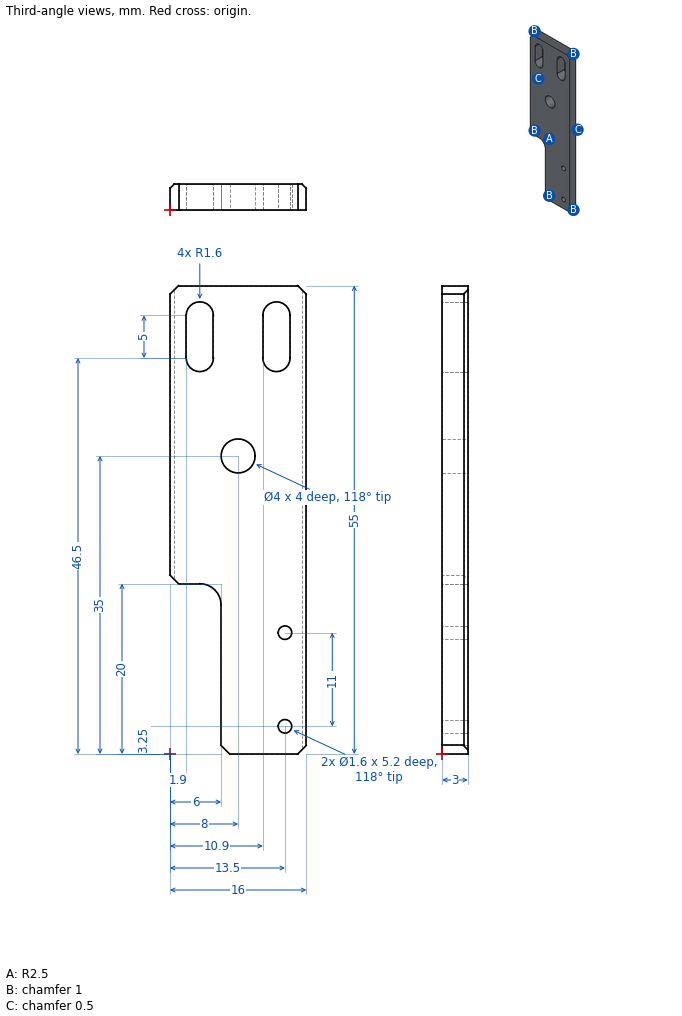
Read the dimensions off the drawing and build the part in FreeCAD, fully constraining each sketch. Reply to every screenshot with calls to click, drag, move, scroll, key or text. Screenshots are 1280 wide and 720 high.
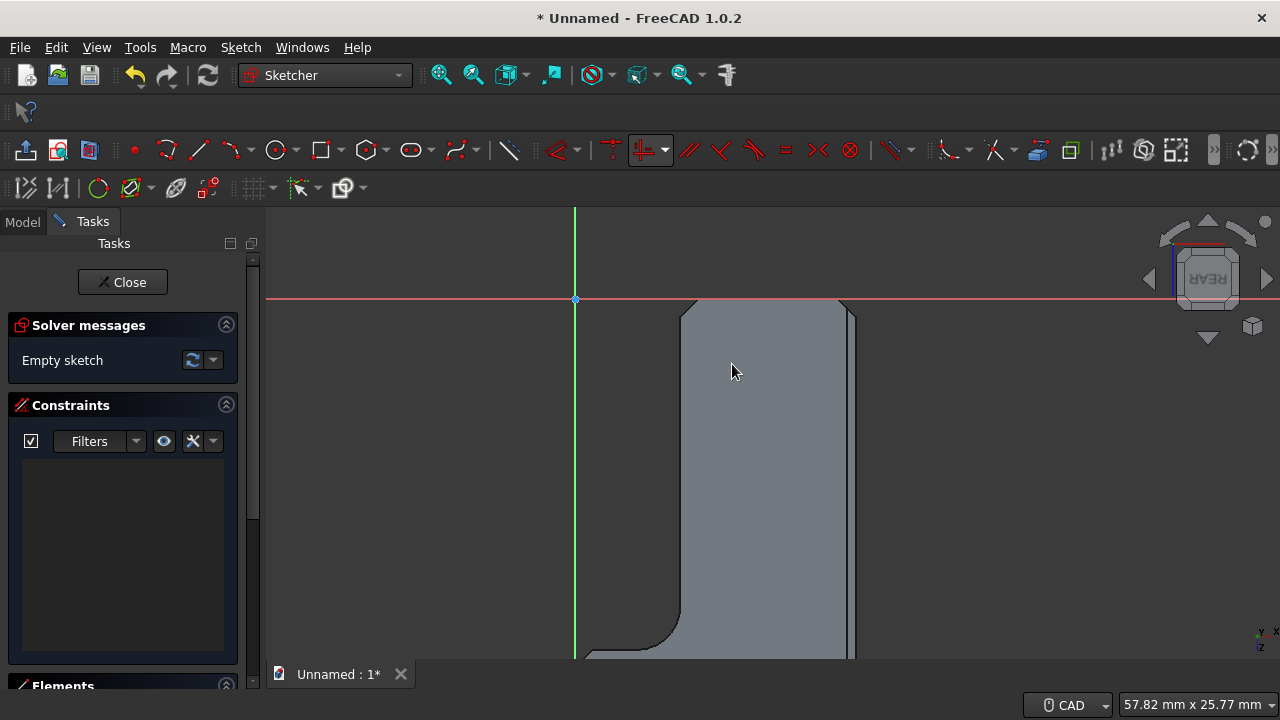
click(276, 150)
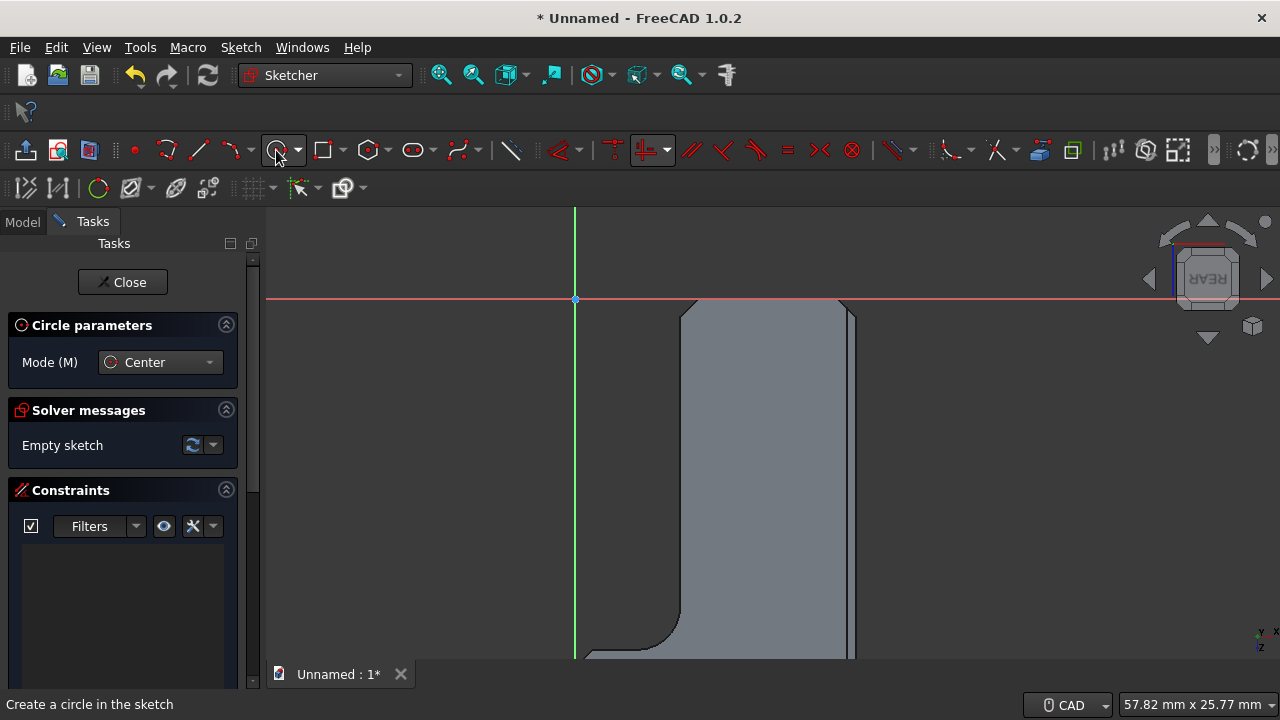
scroll(812, 356, up, 3)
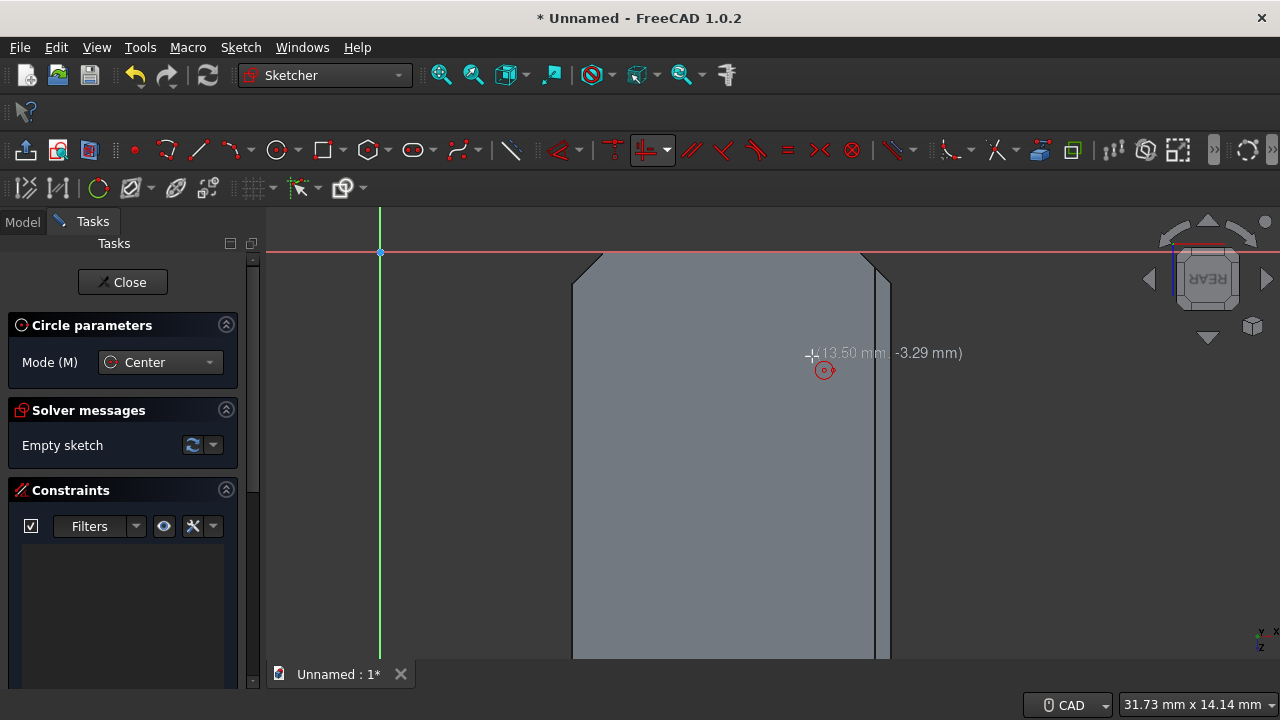
click(811, 356)
move(830, 338)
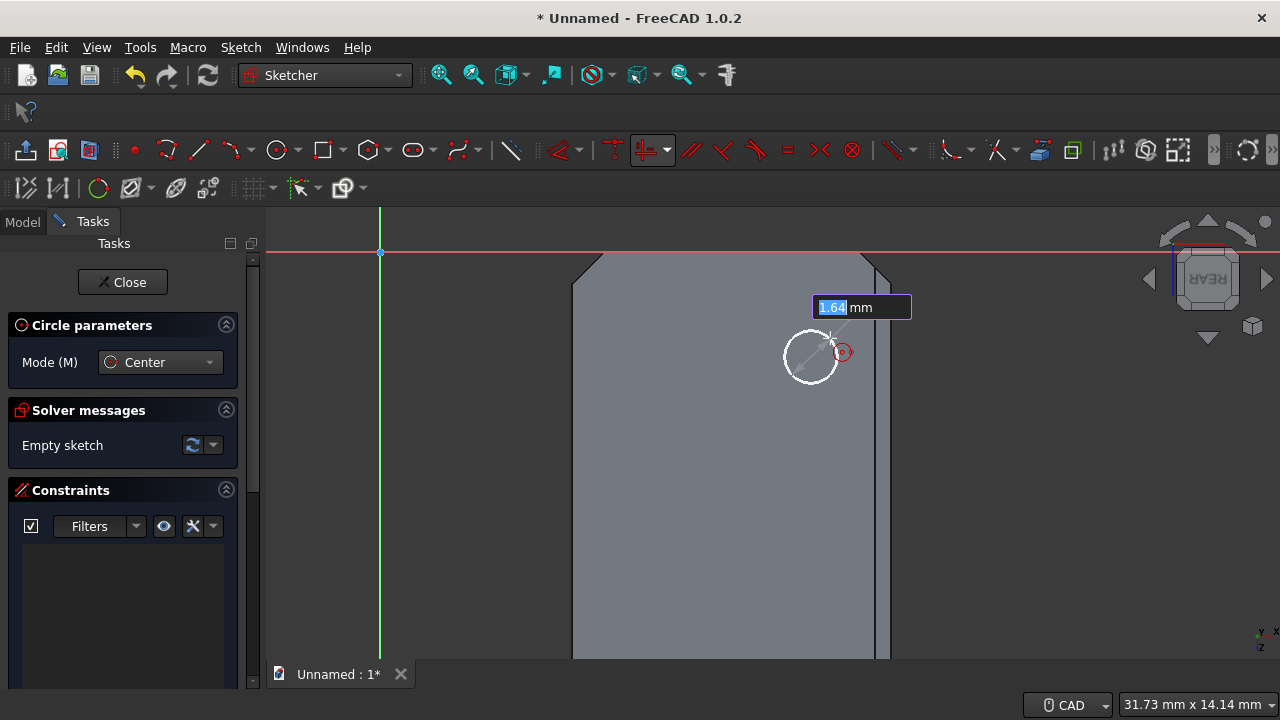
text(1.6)
key(Return)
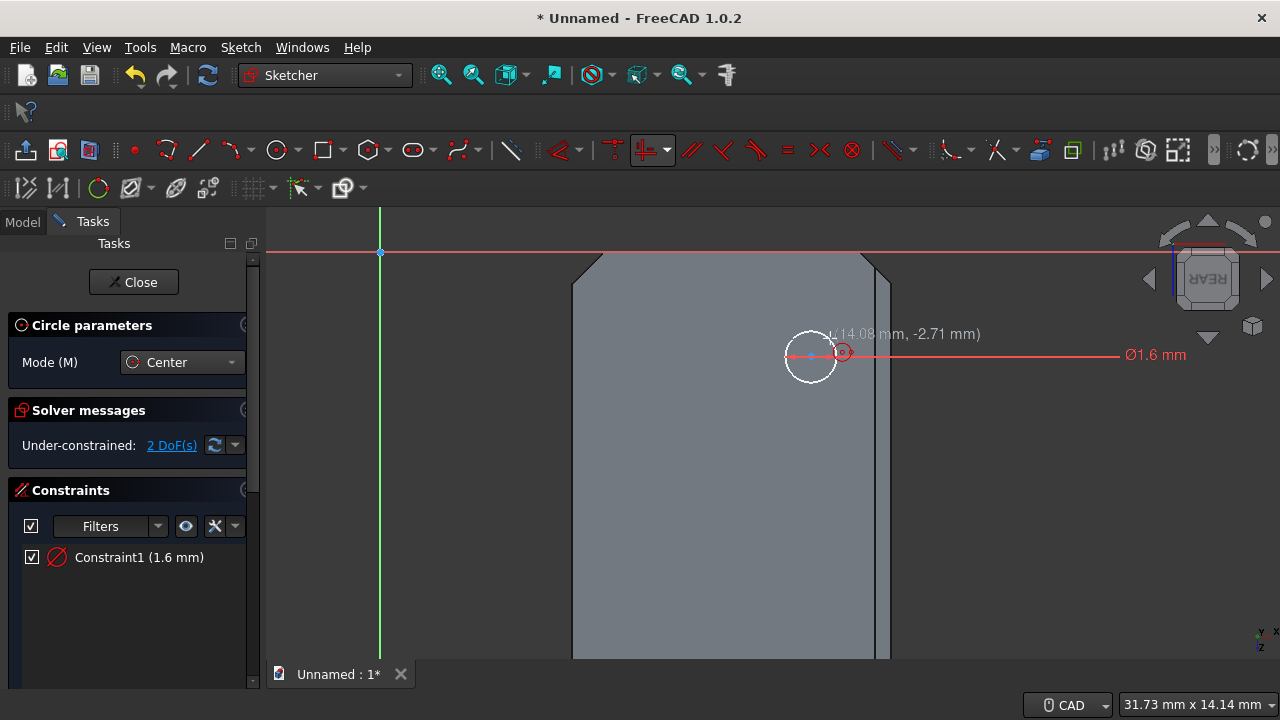
scroll(821, 360, down, 3)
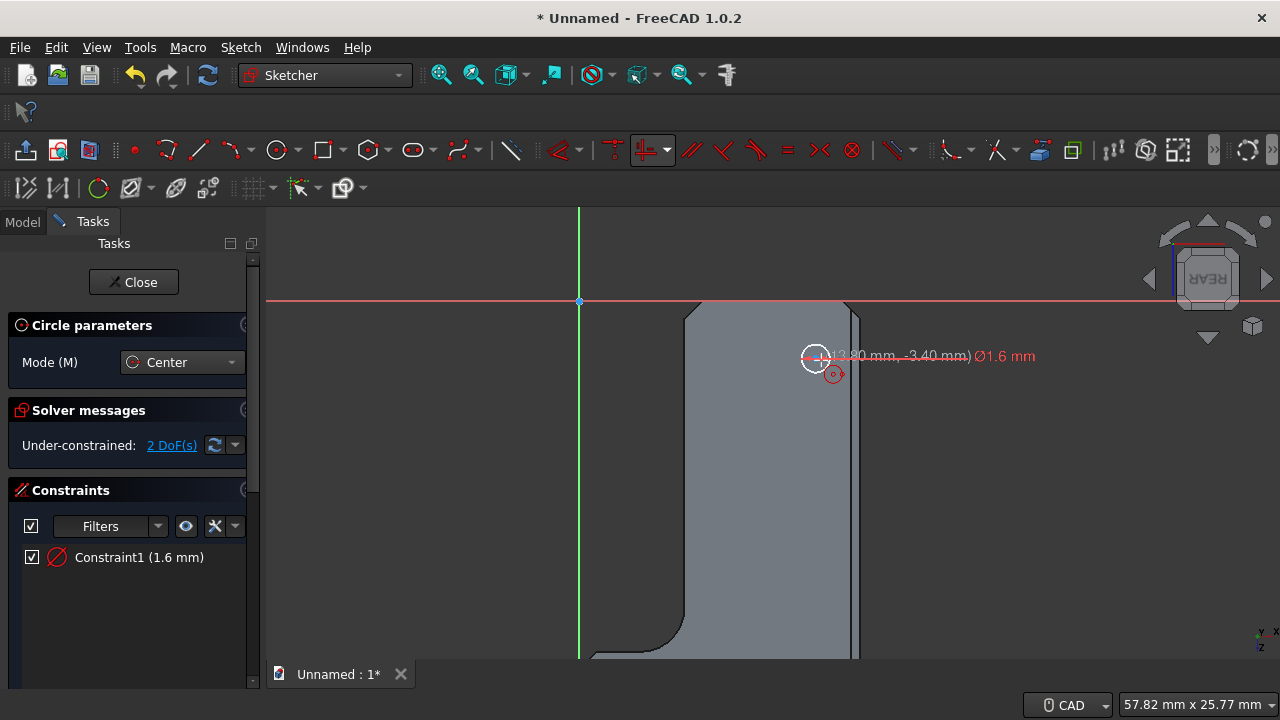
scroll(816, 551, up, 3)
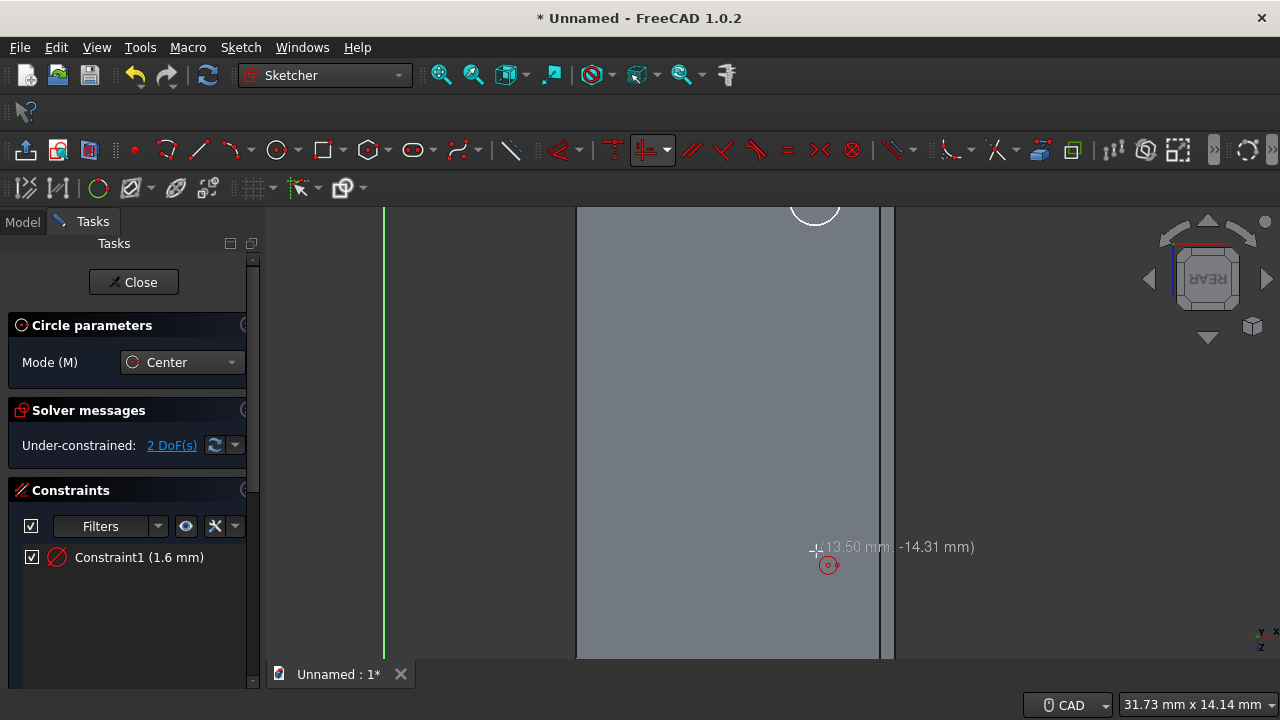
click(816, 550)
move(834, 532)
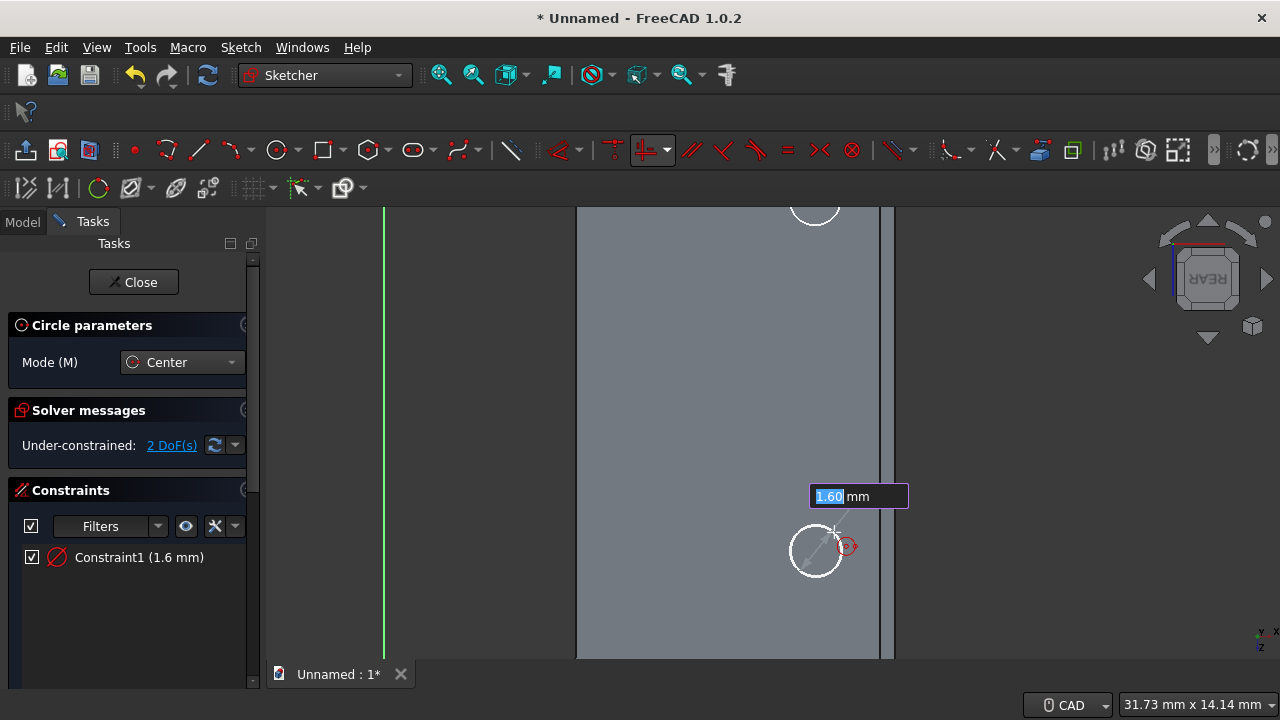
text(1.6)
key(Return)
key(Escape)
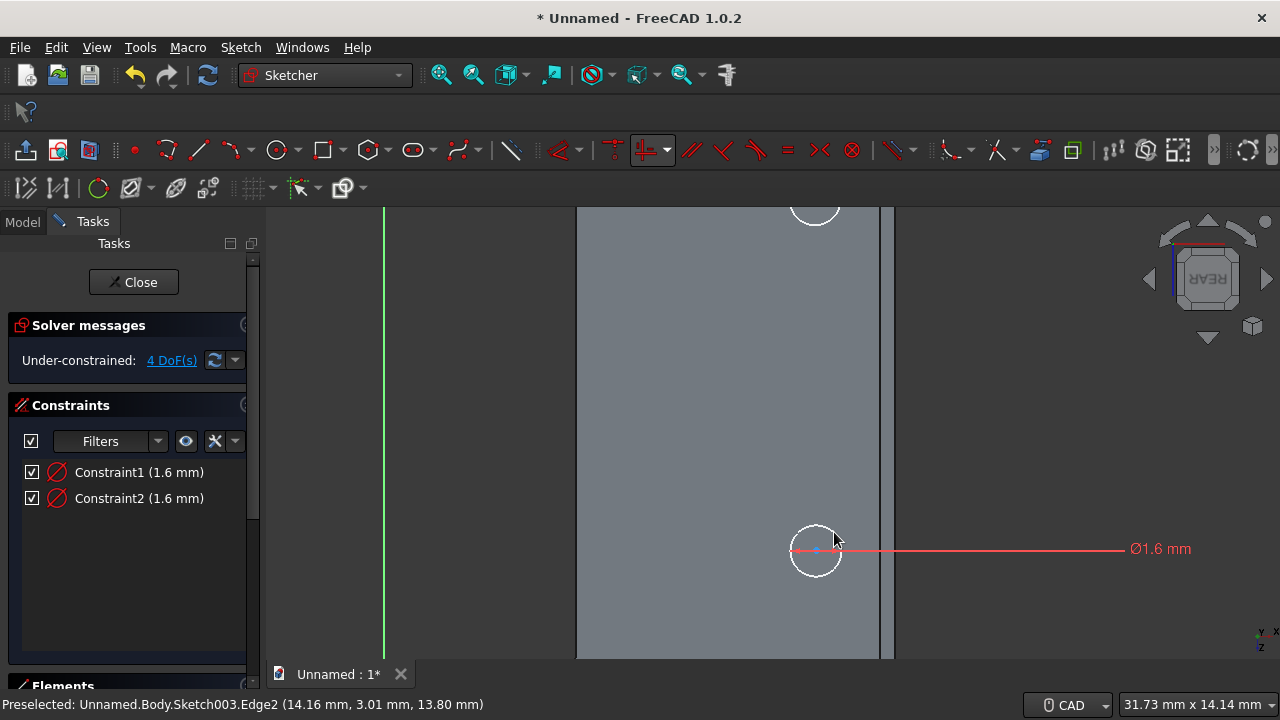
click(558, 150)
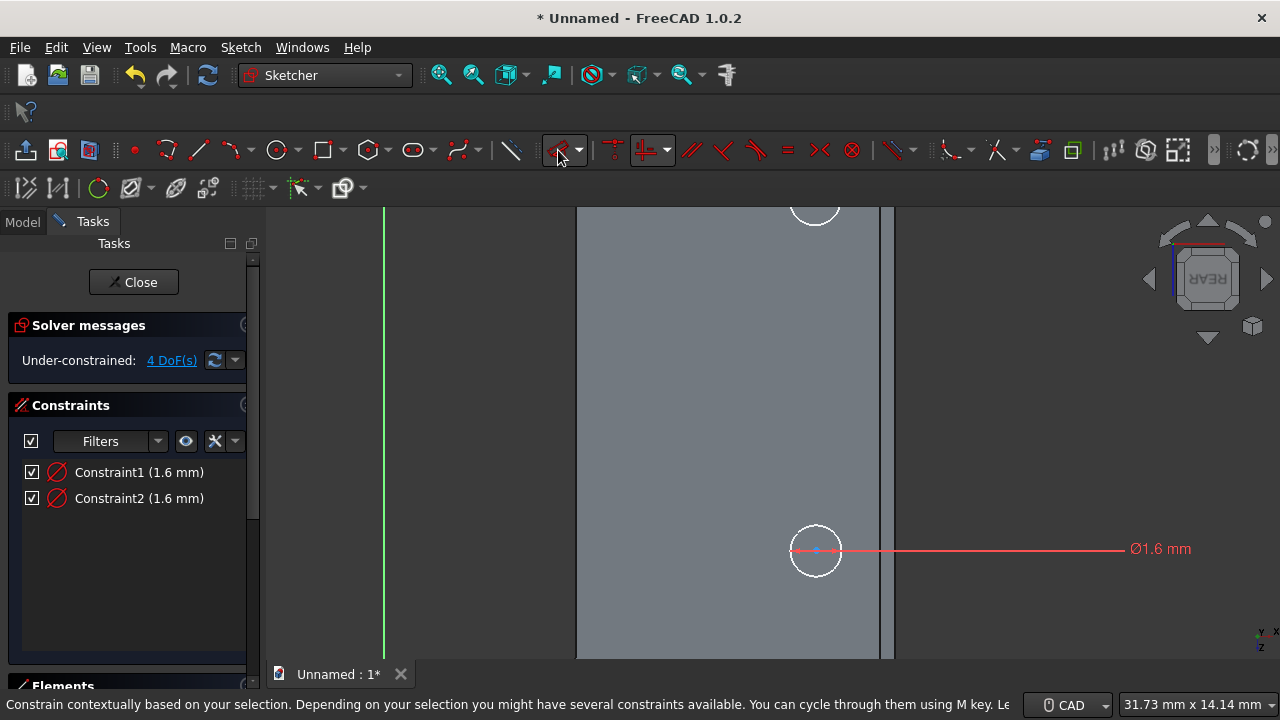
scroll(816, 552, down, 3)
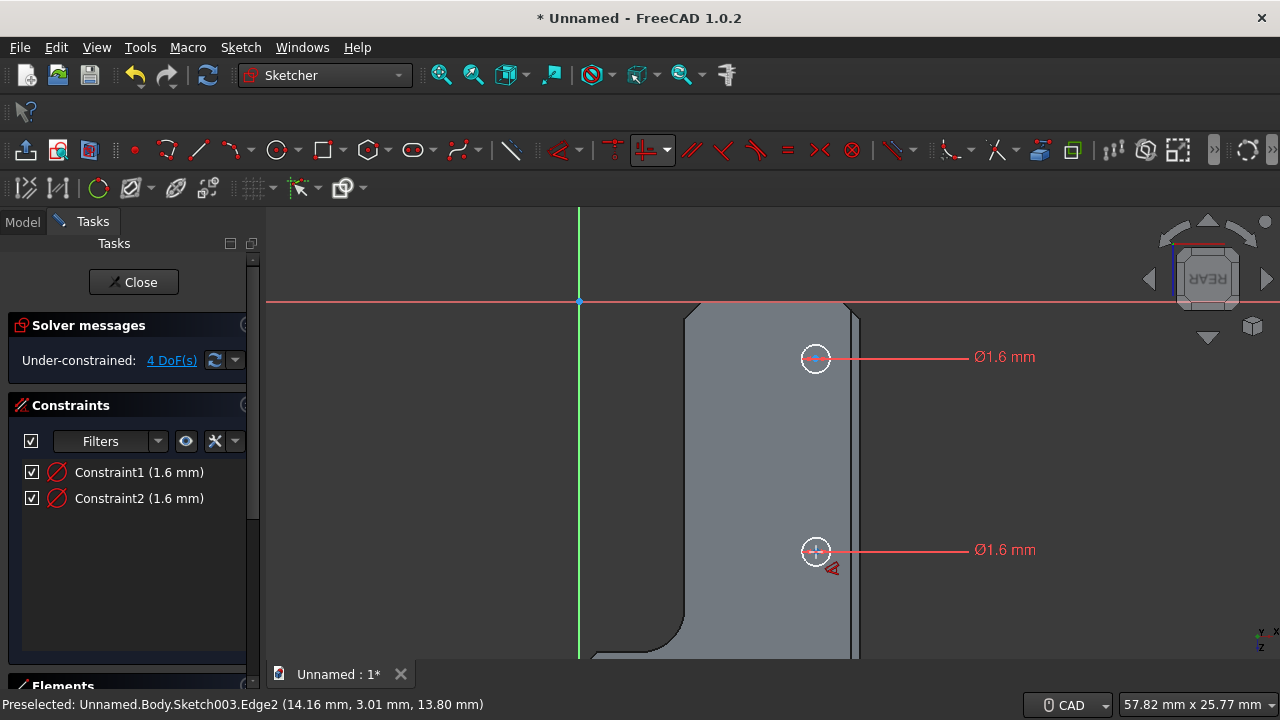
click(816, 359)